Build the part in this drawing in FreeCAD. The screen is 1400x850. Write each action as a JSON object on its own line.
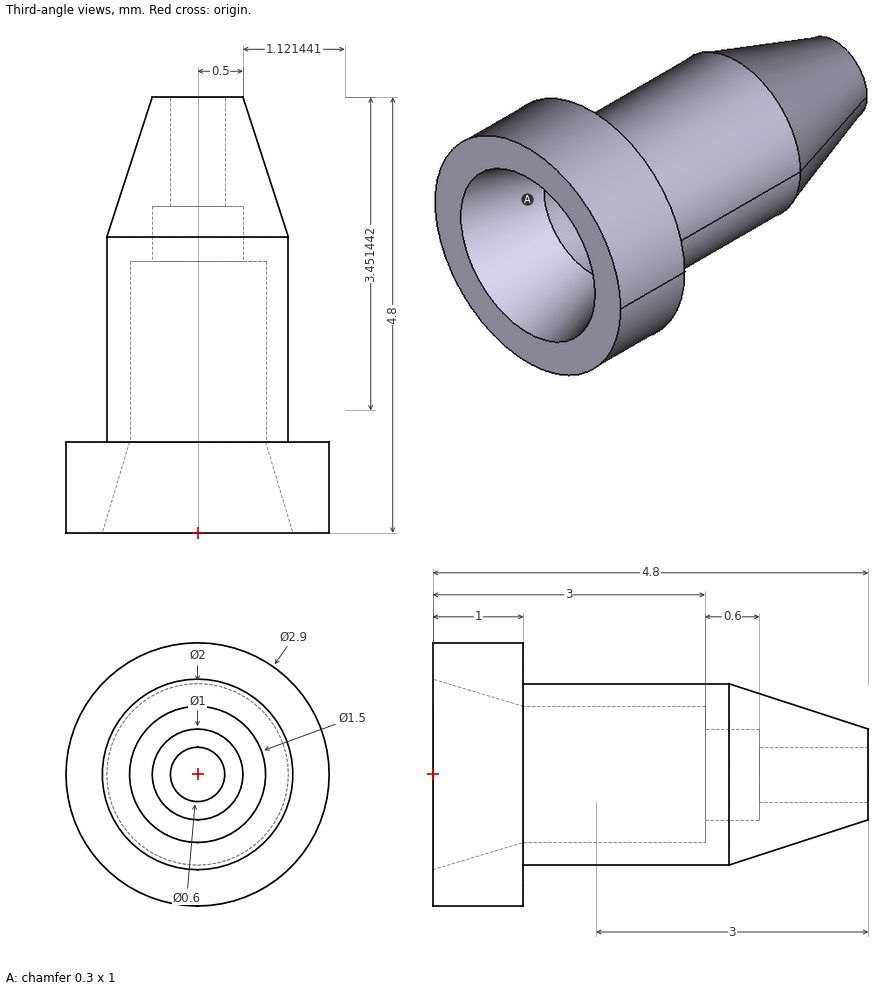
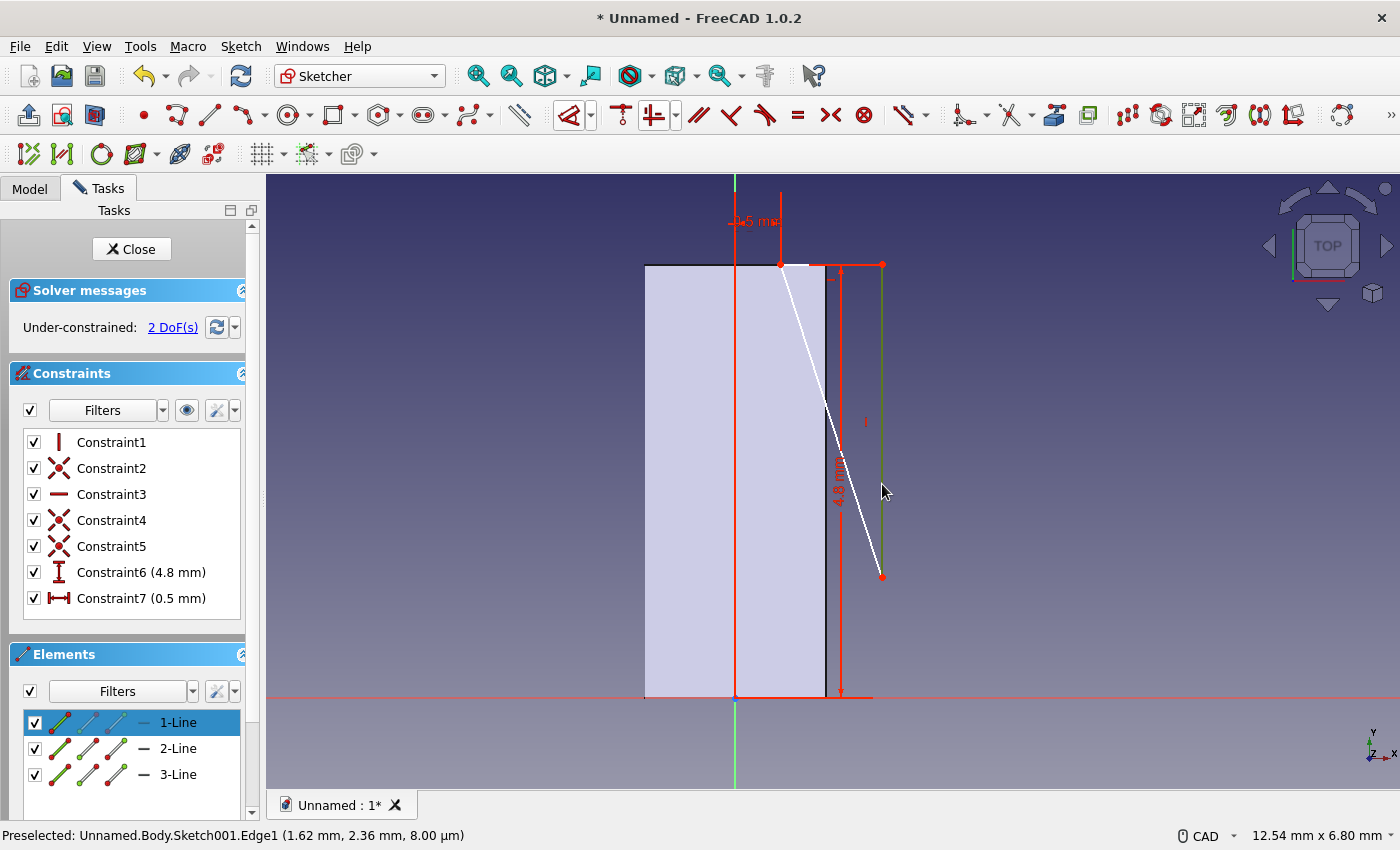
{"action": "key", "text": "i"}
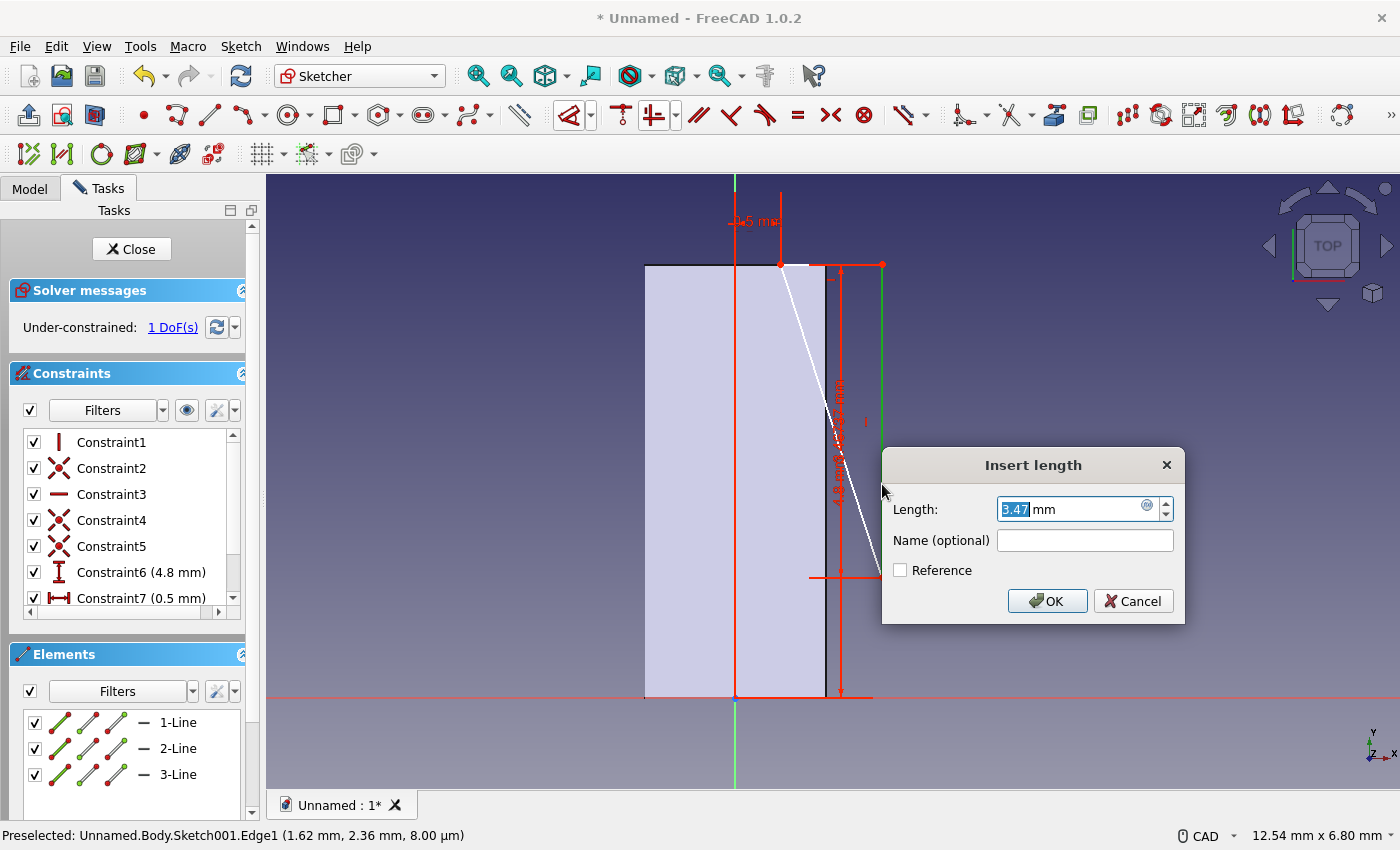
{"action": "type", "text": "3.451442"}
{"action": "key", "text": "Return"}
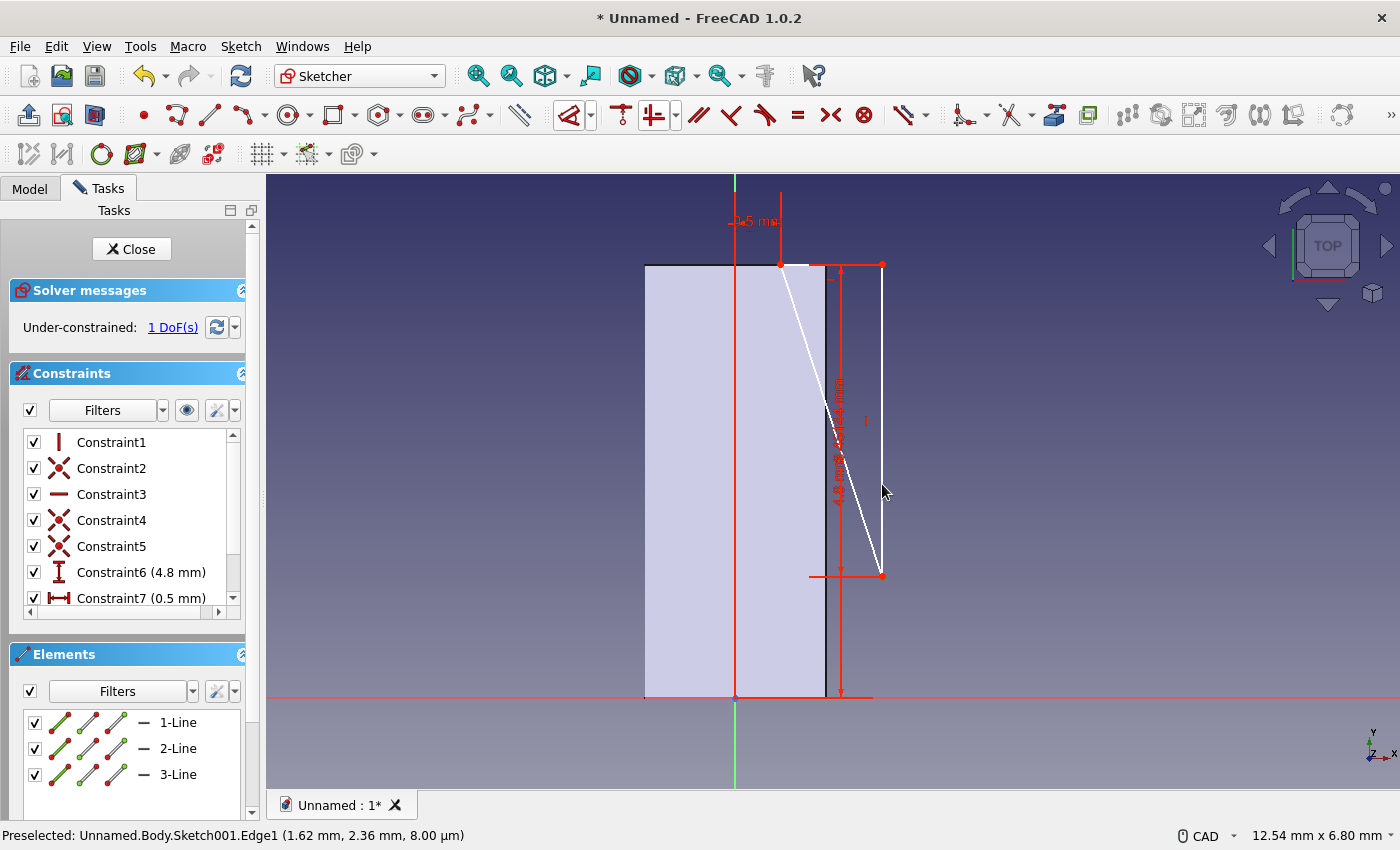
{"action": "left_click", "coordinate": [852, 265]}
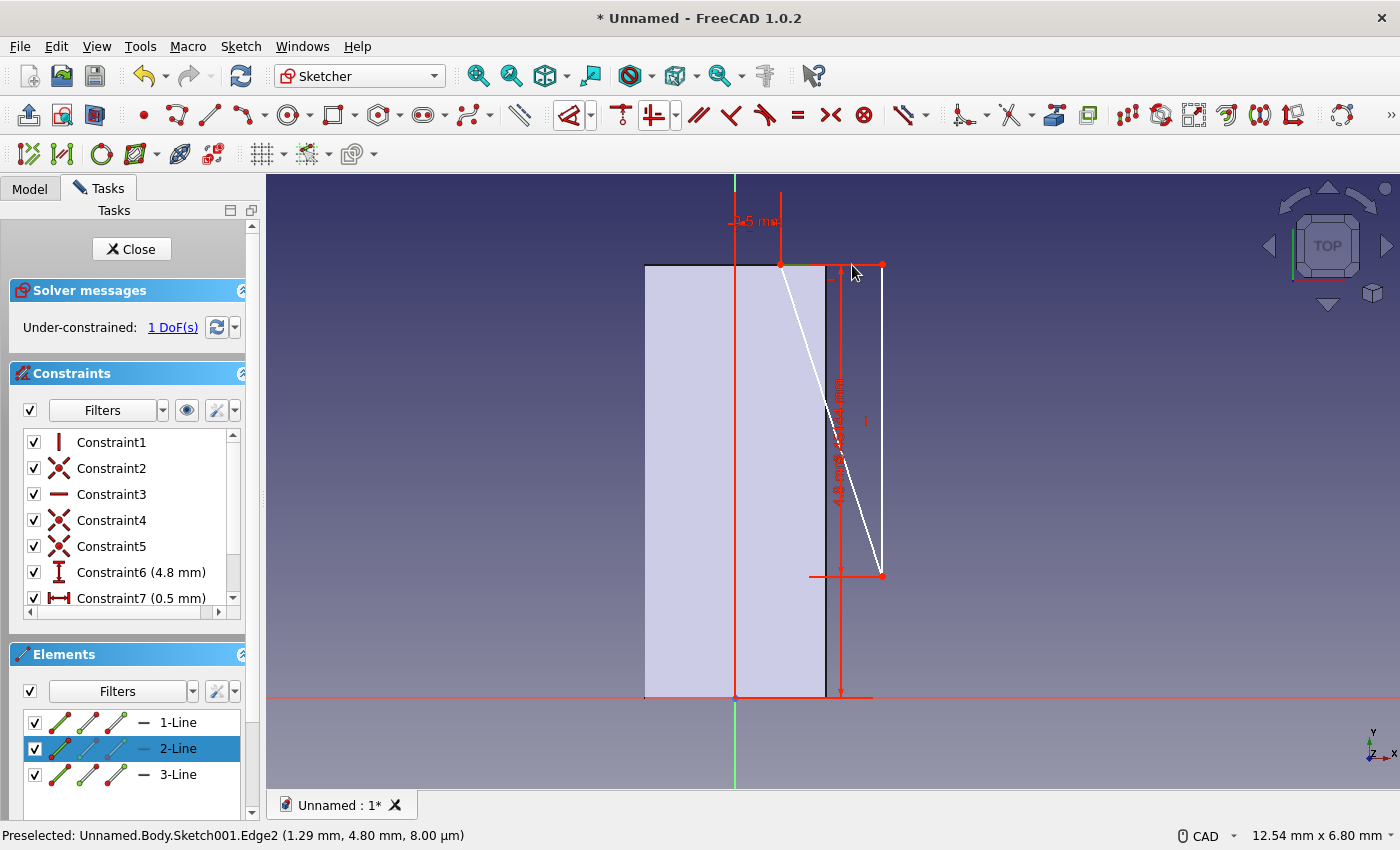
{"action": "key", "text": "l"}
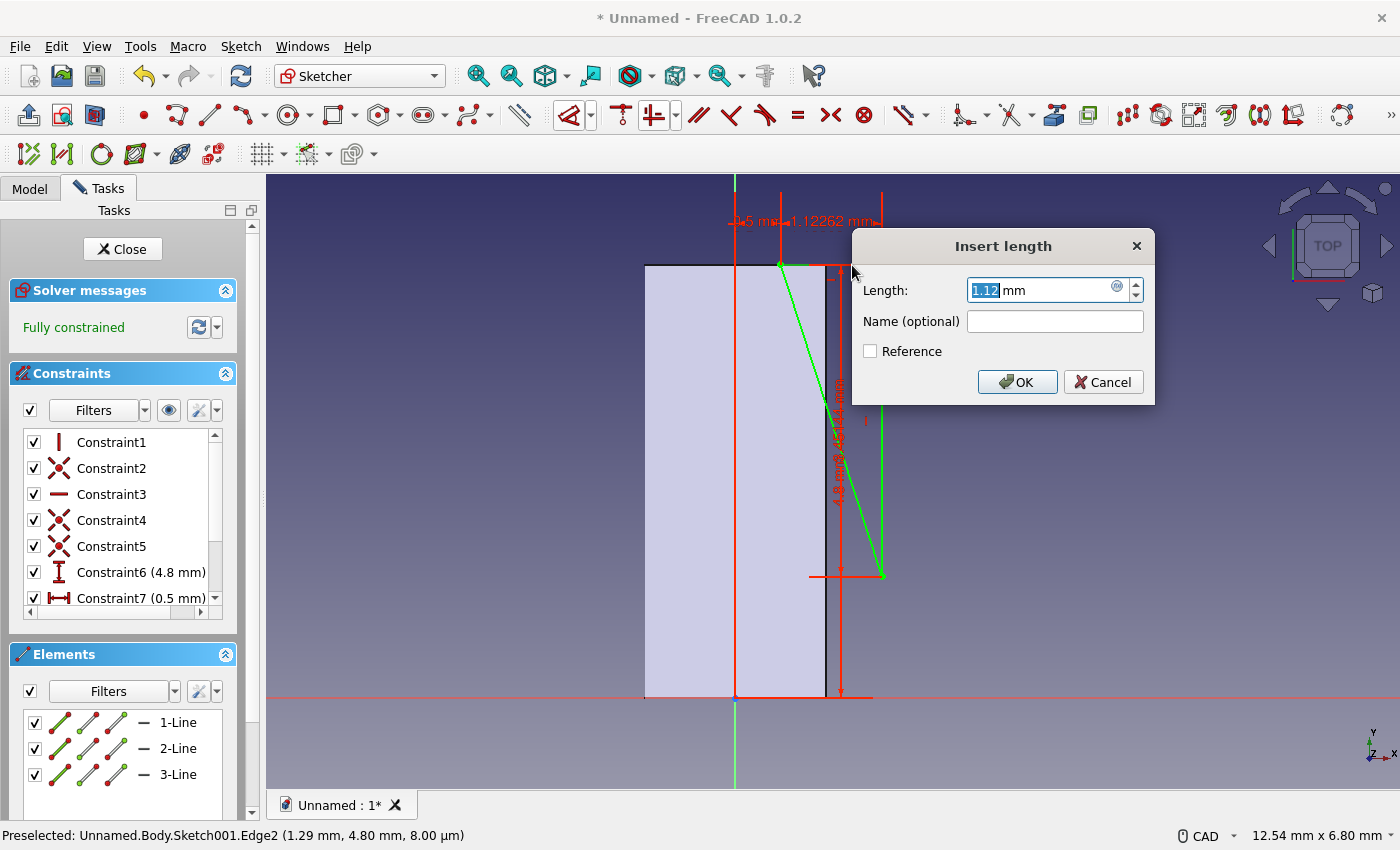
{"action": "type", "text": "1.121441"}
{"action": "key", "text": "Return"}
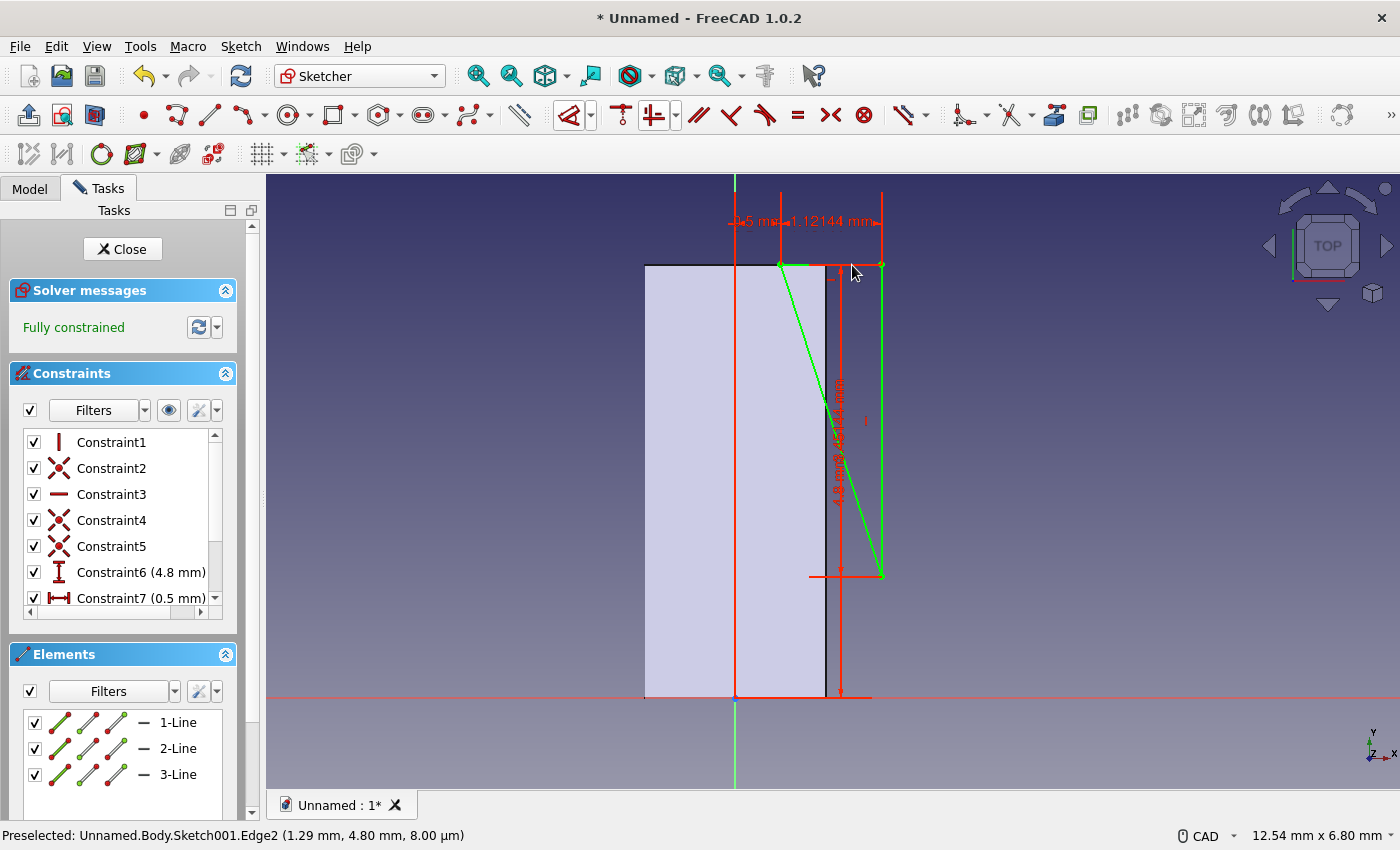
{"action": "left_click", "coordinate": [123, 249]}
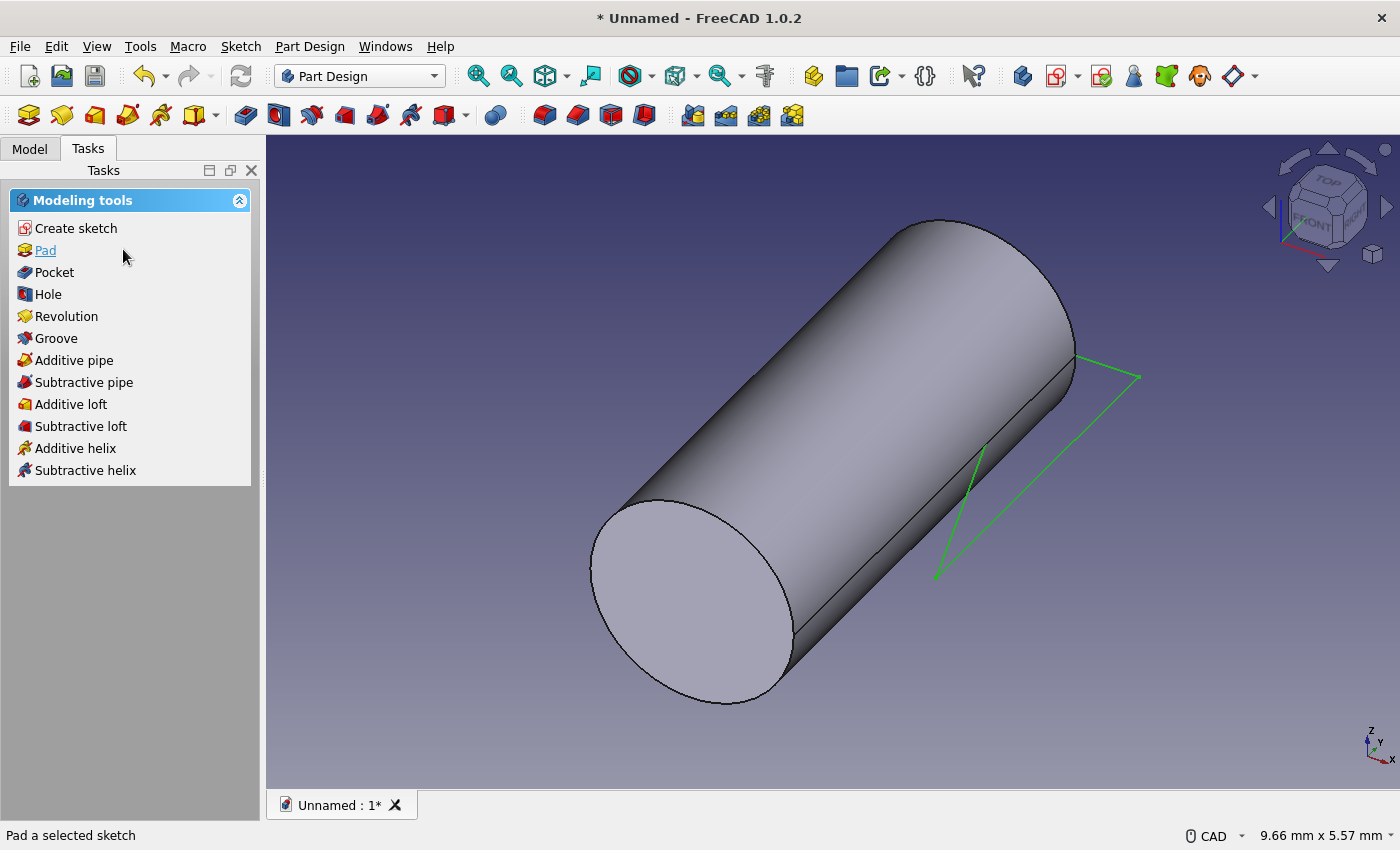
{"action": "left_click", "coordinate": [312, 116]}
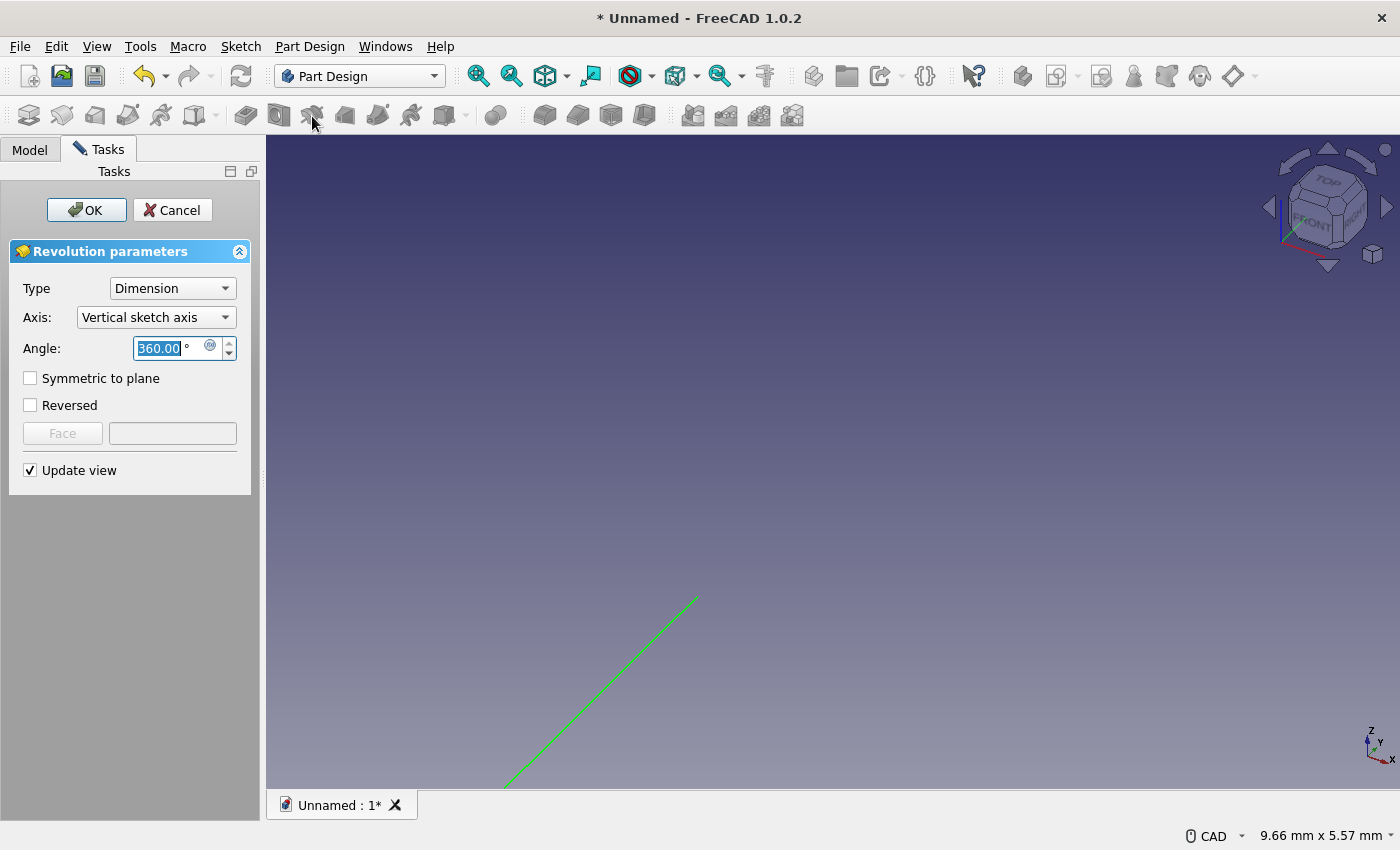
{"action": "left_click", "coordinate": [87, 210]}